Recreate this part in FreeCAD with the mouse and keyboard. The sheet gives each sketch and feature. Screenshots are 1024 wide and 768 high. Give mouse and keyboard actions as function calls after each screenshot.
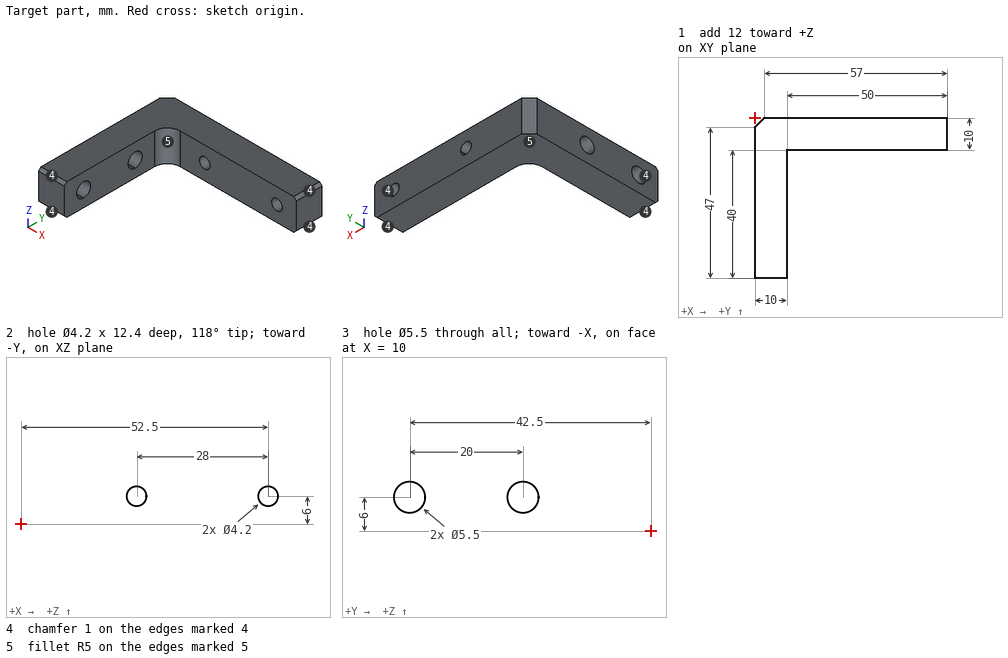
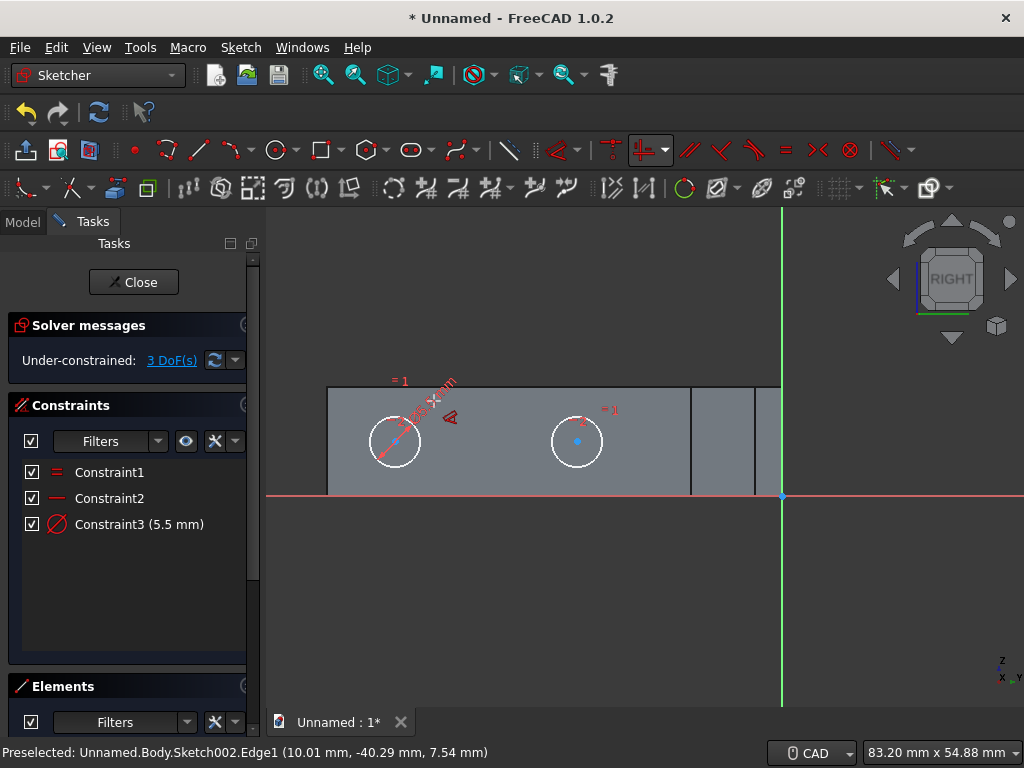
click(395, 442)
click(816, 469)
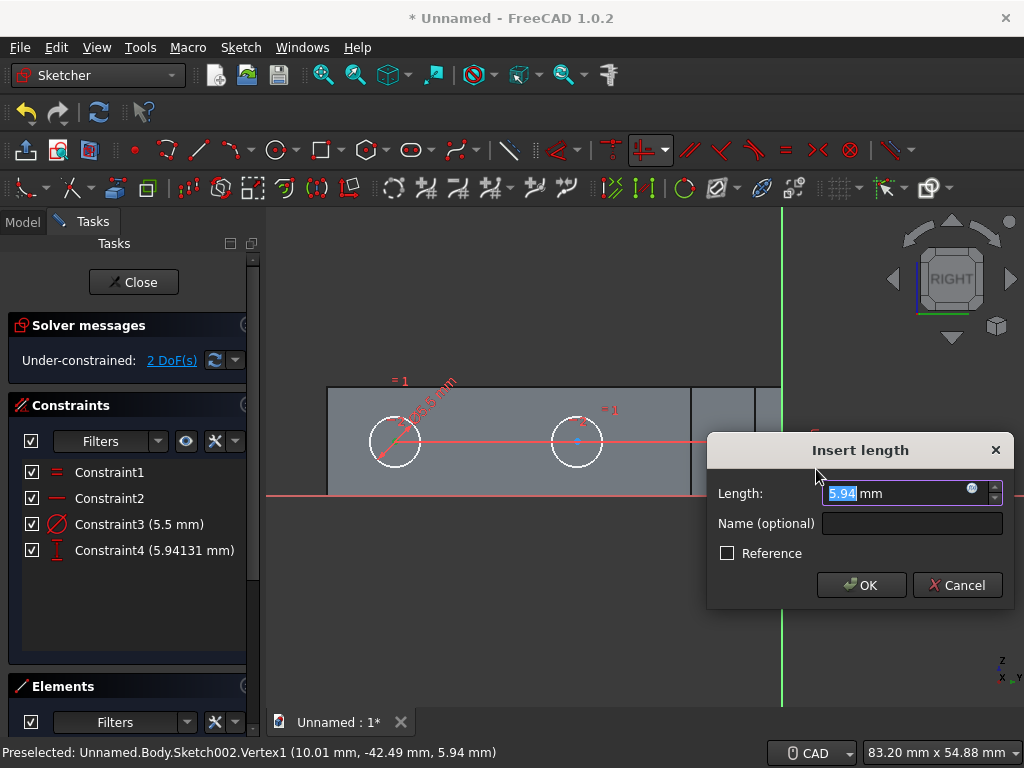
text(6)
key(Return)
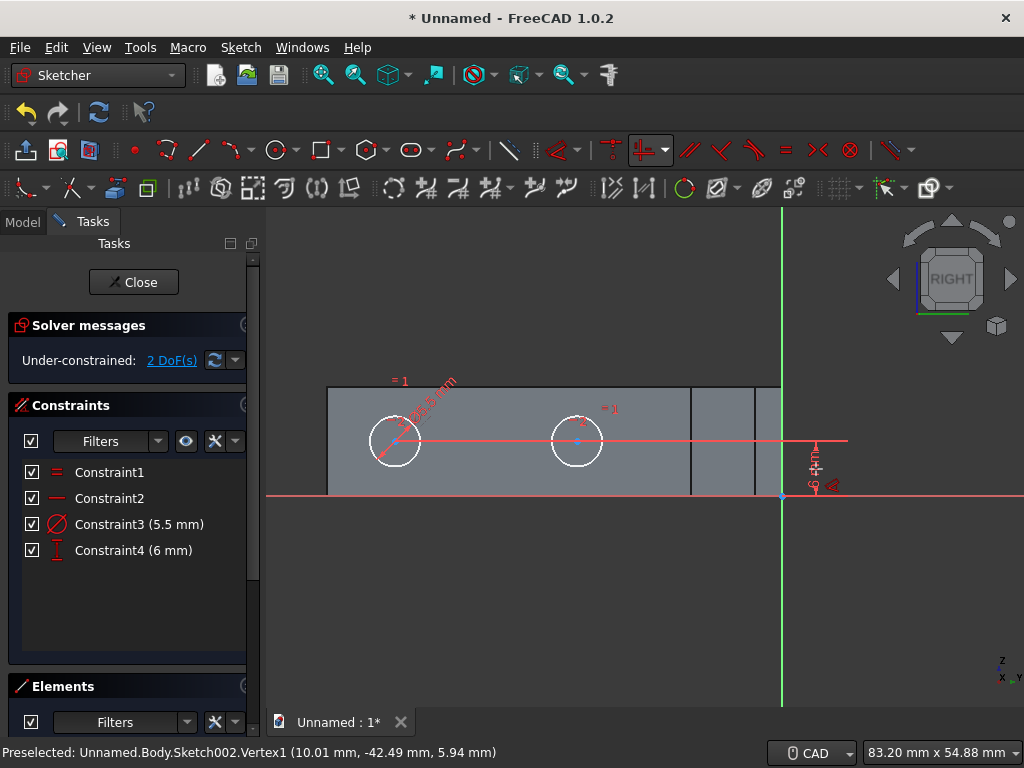
click(395, 441)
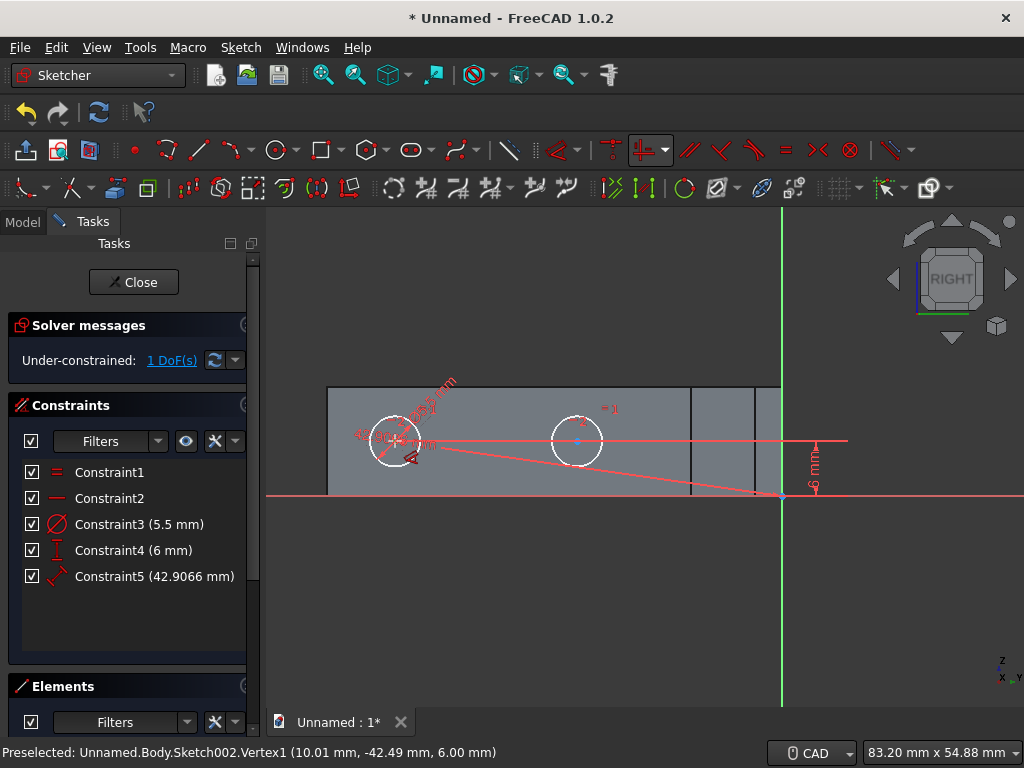
click(577, 441)
click(528, 407)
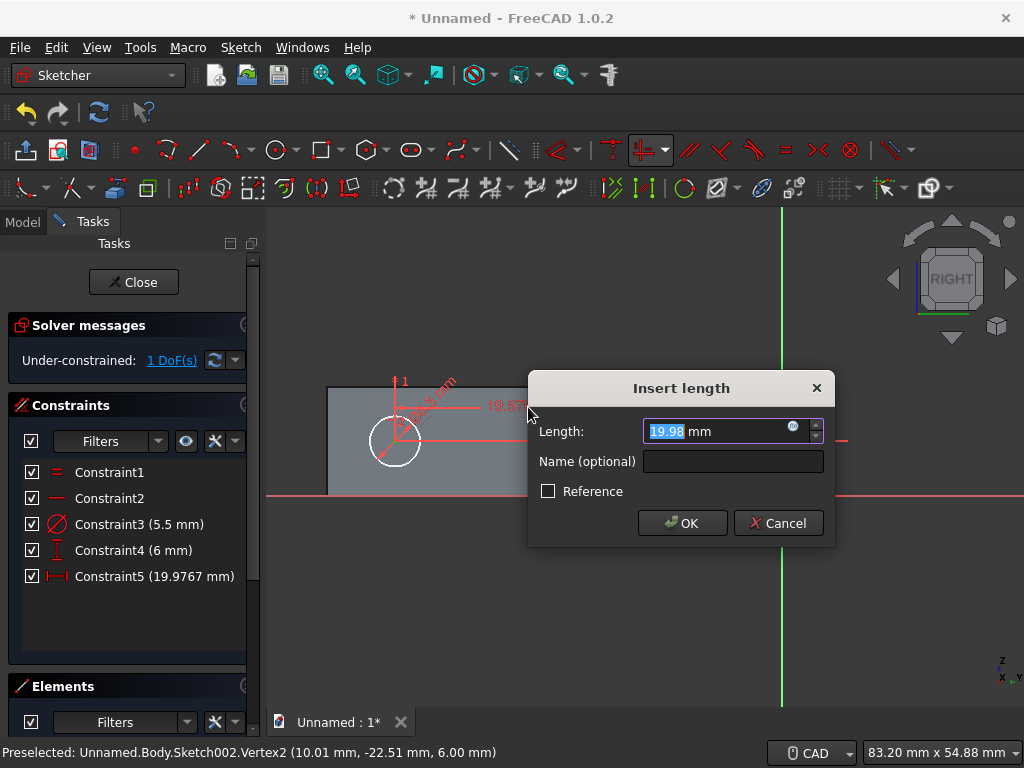
text(20)
key(Return)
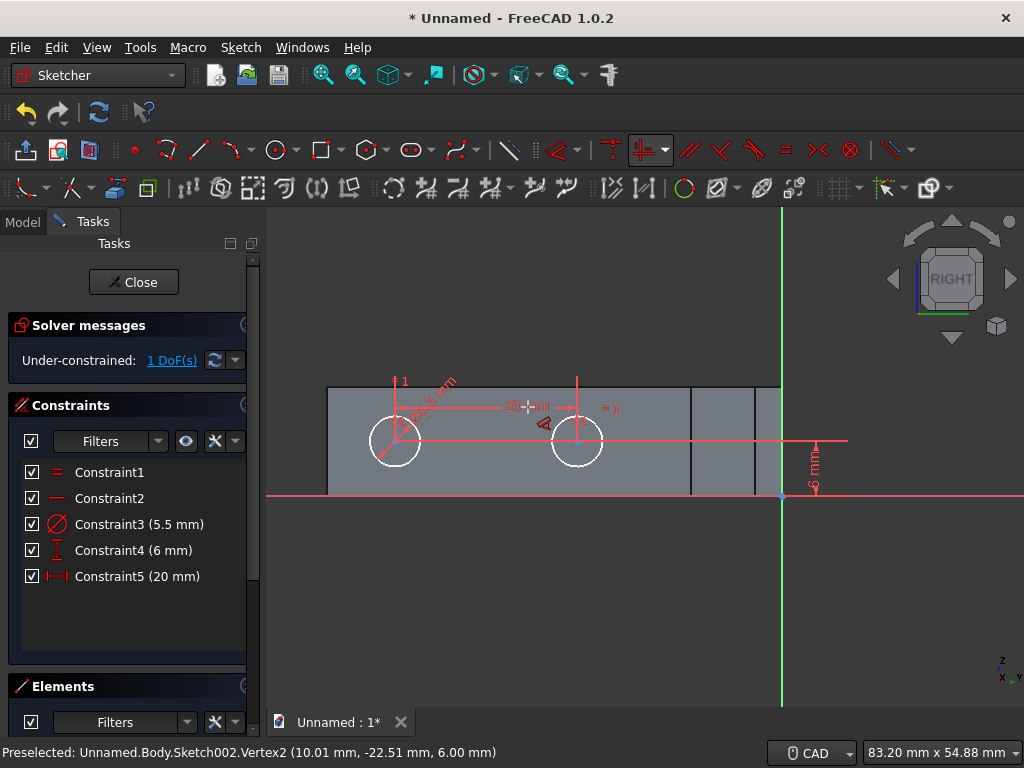
click(395, 441)
click(589, 530)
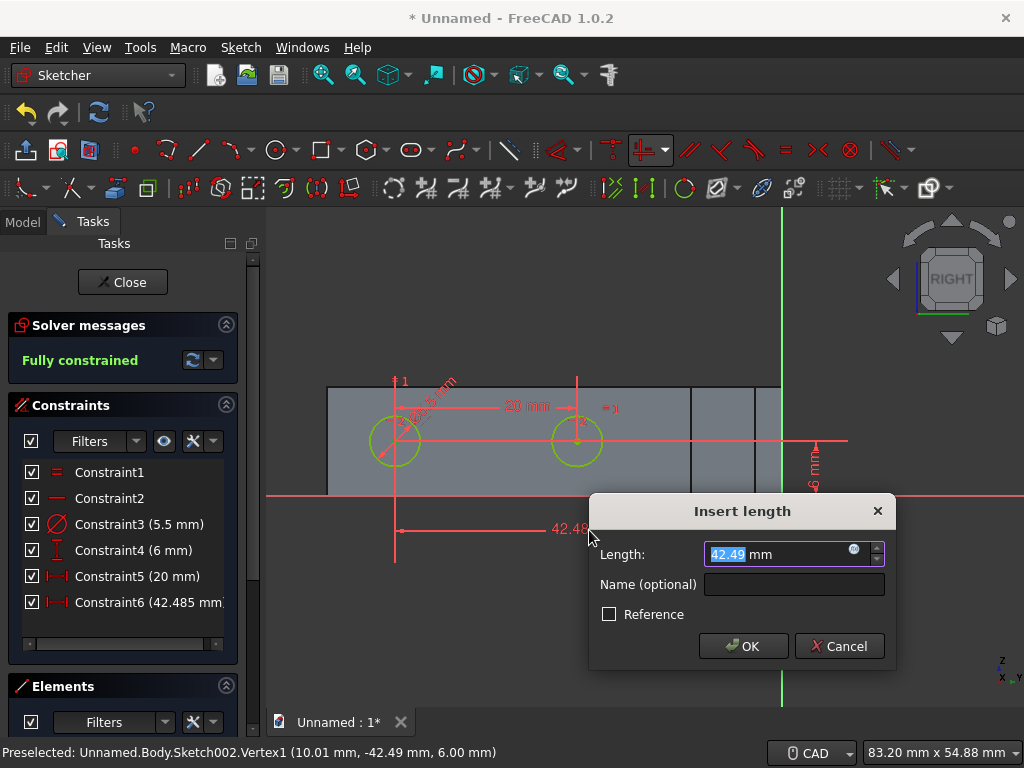
text(42.5)
key(Return)
key(Escape)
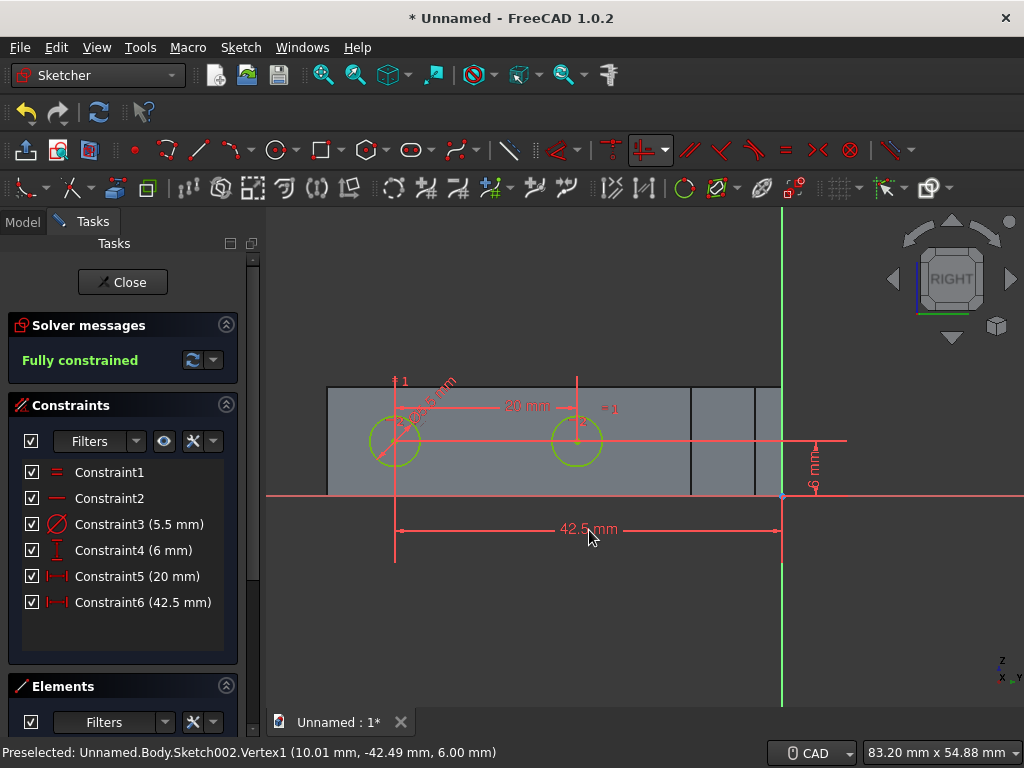
click(123, 282)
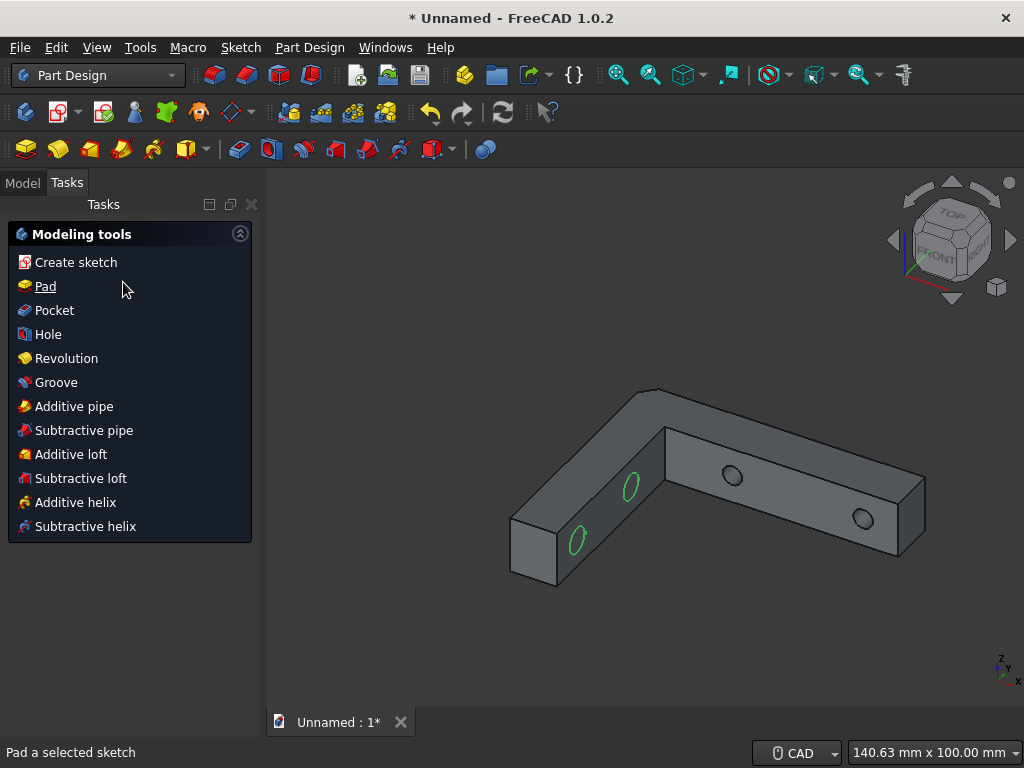
click(272, 150)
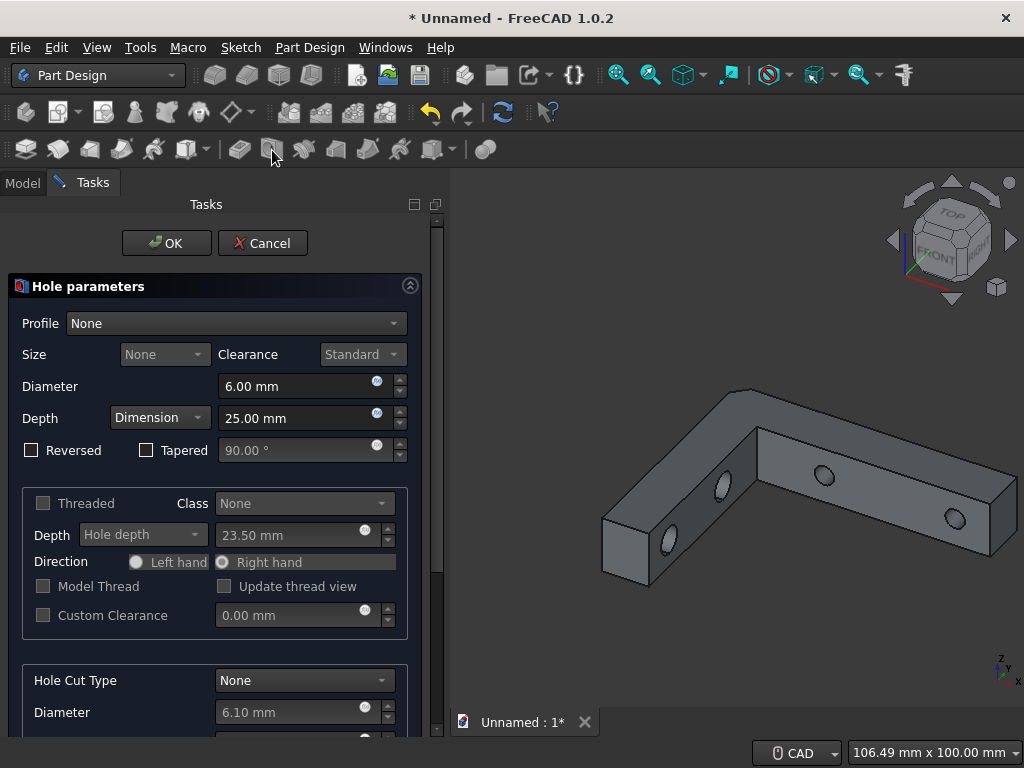
triple_click(305, 386)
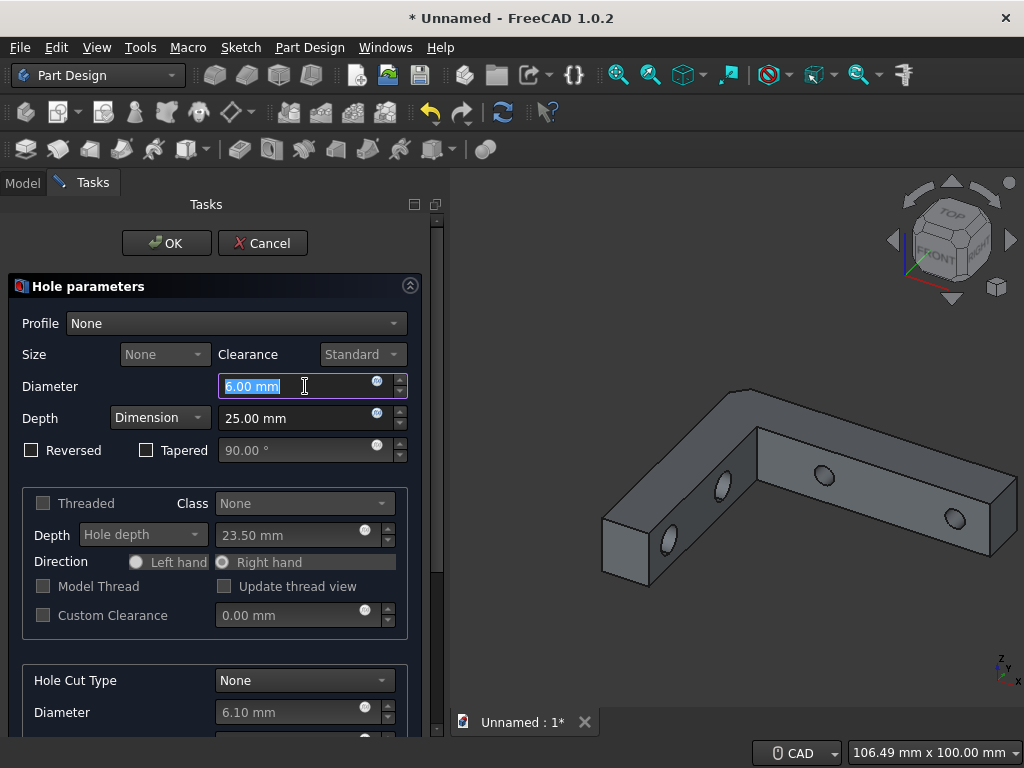
text(5.5)
key(Tab)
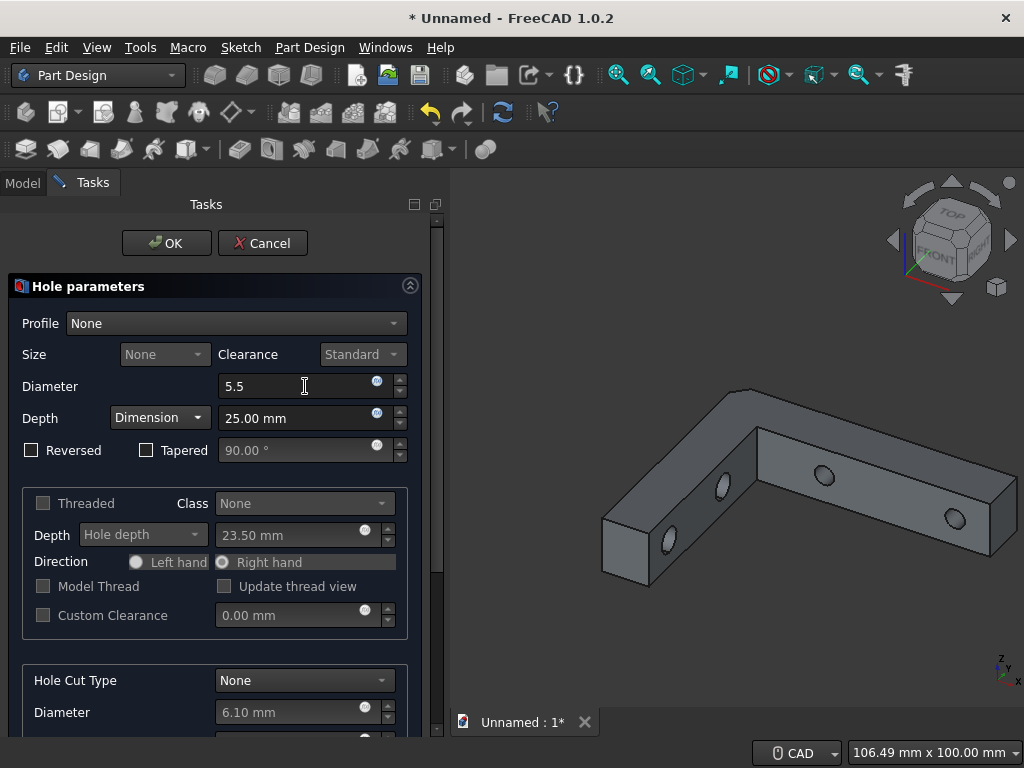
click(161, 418)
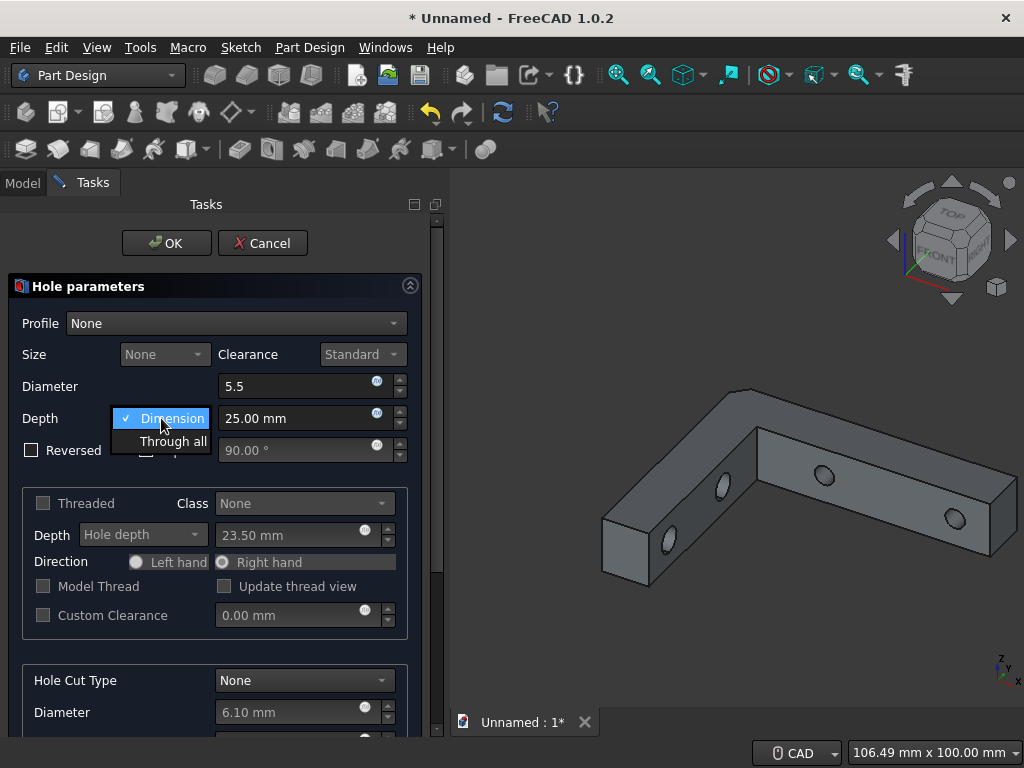
click(160, 442)